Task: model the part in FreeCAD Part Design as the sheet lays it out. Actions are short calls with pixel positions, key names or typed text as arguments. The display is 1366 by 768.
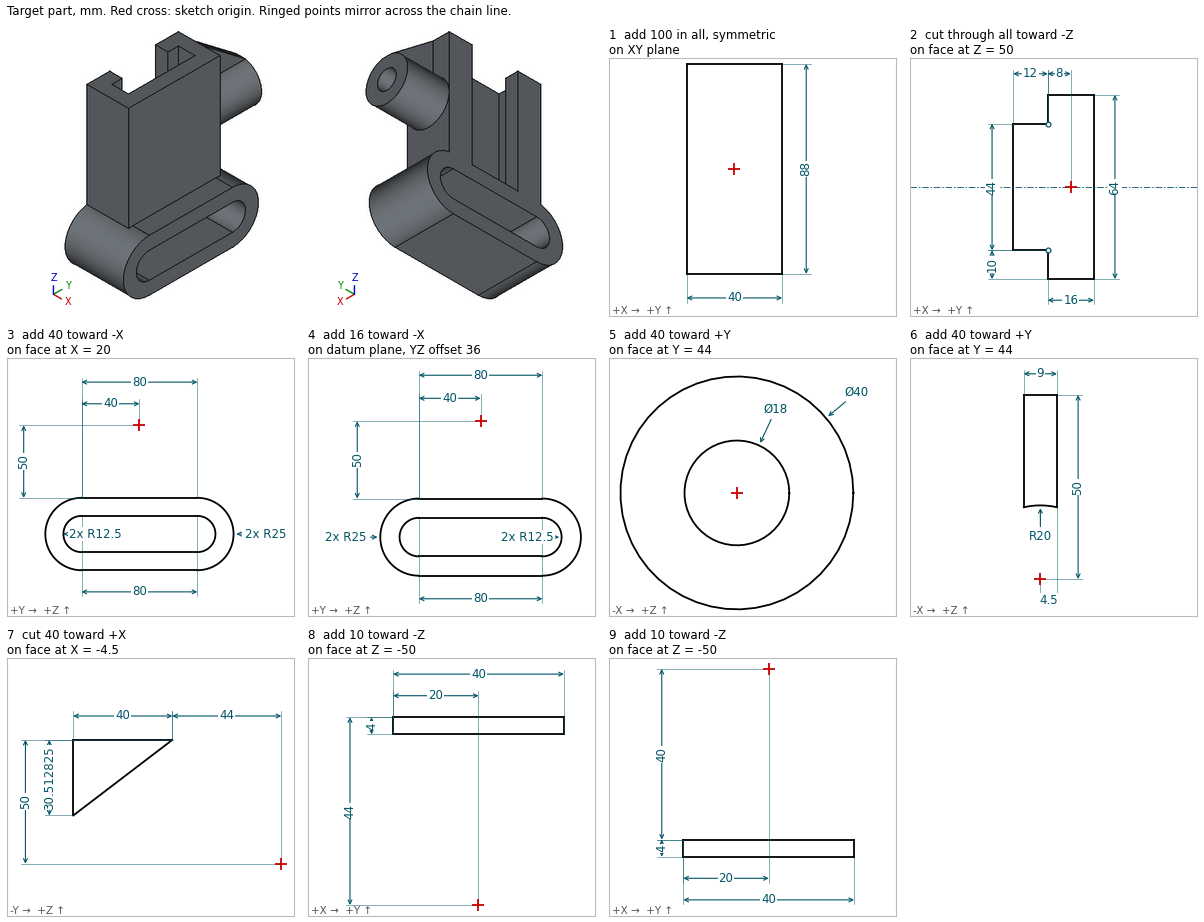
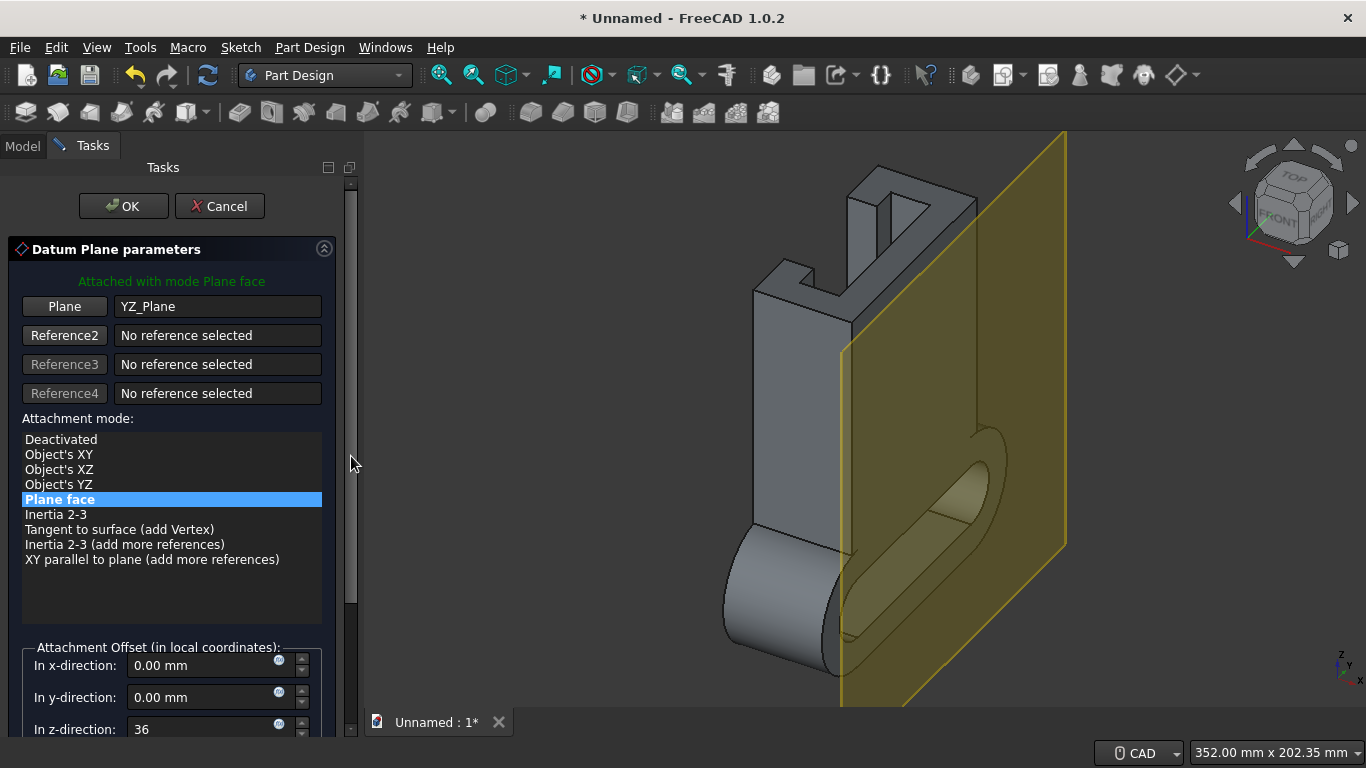
click(124, 206)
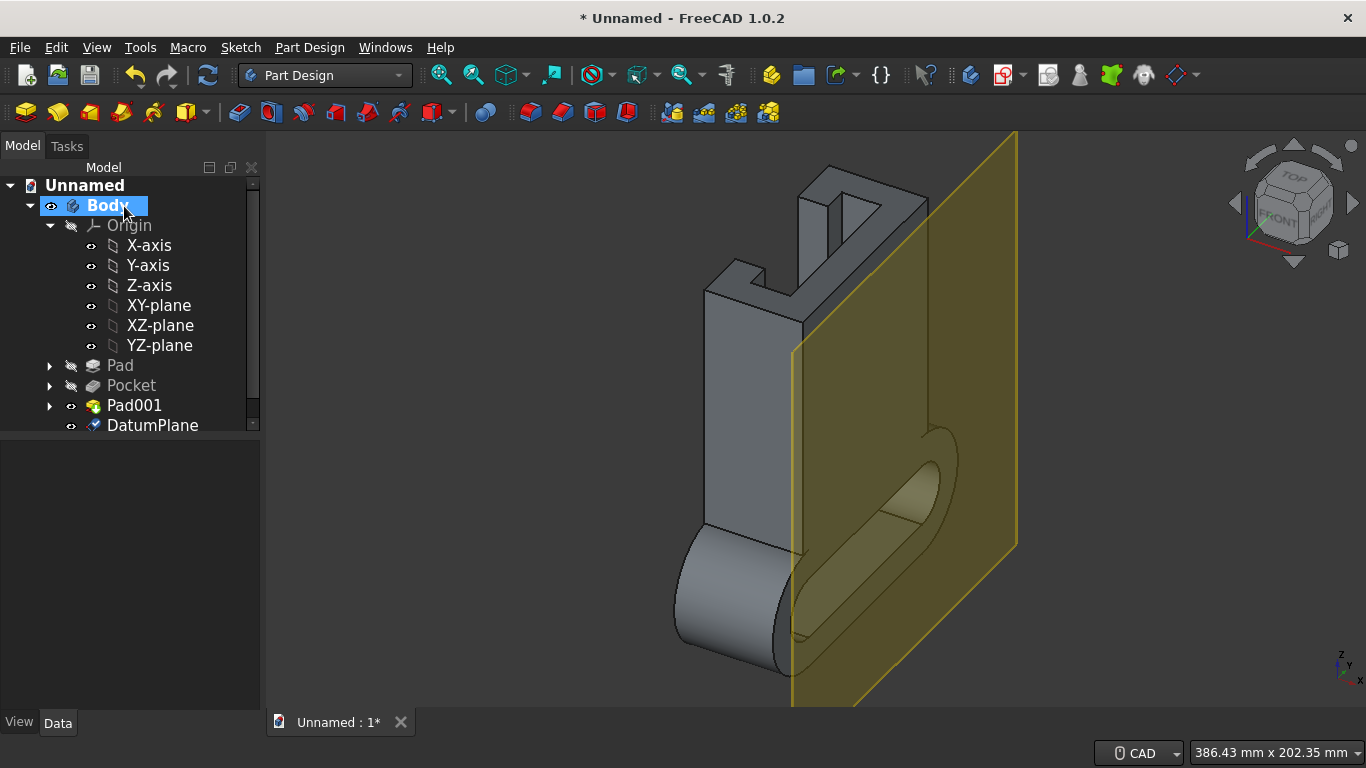
click(116, 426)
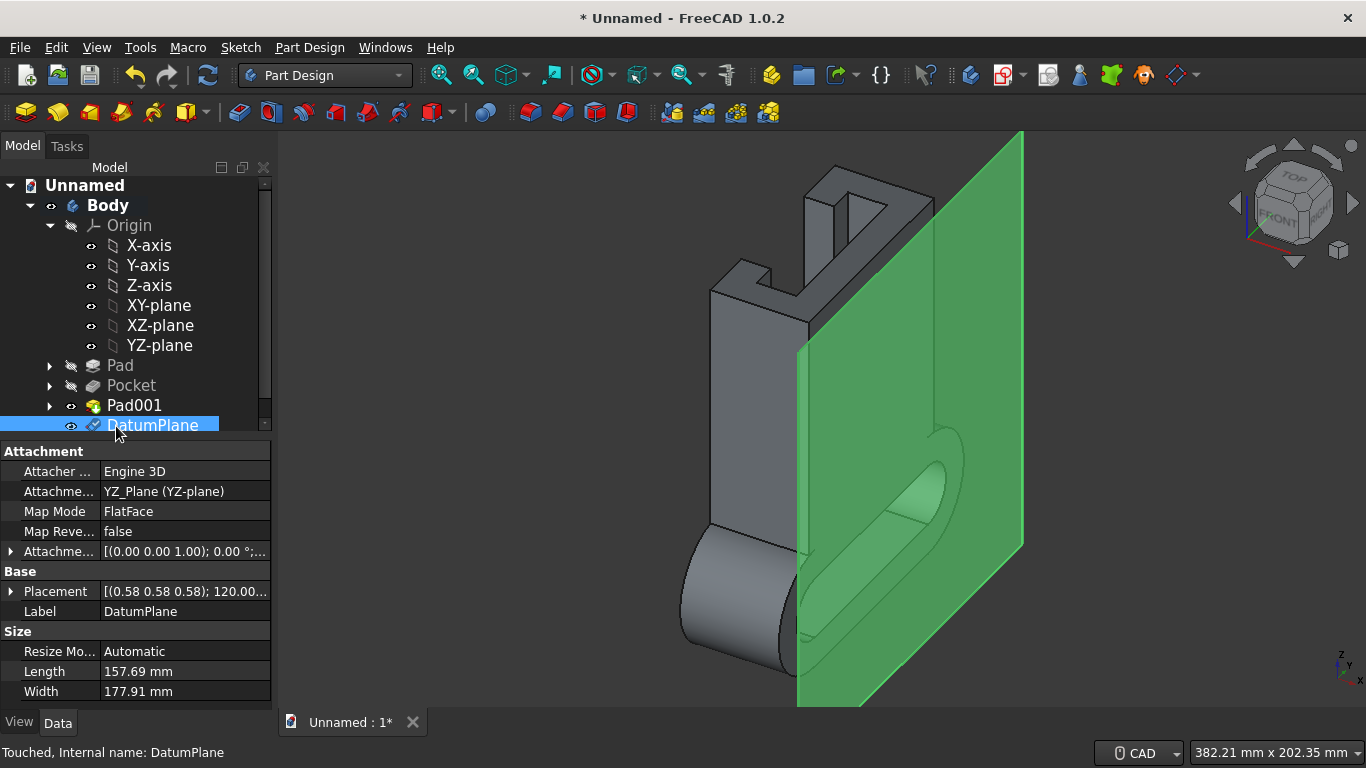
click(1004, 76)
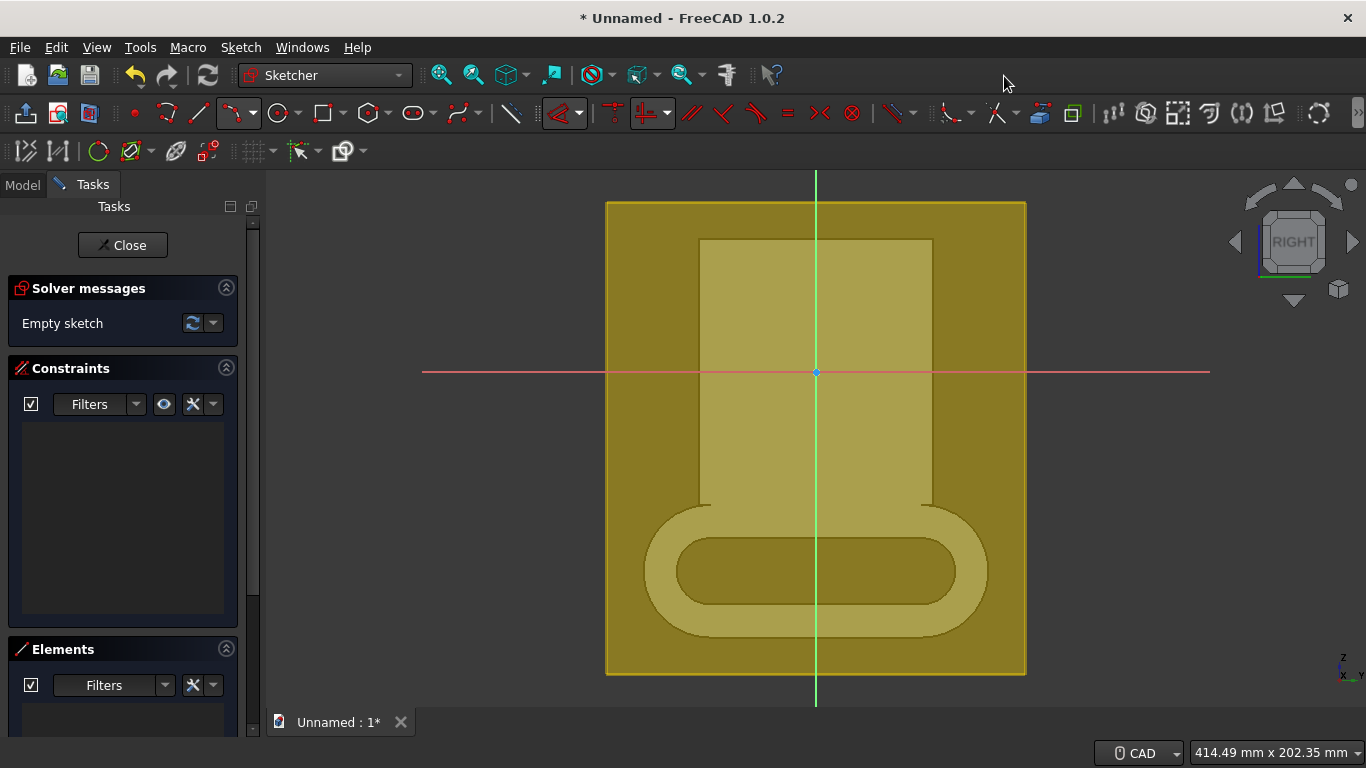
key(g)
key(s)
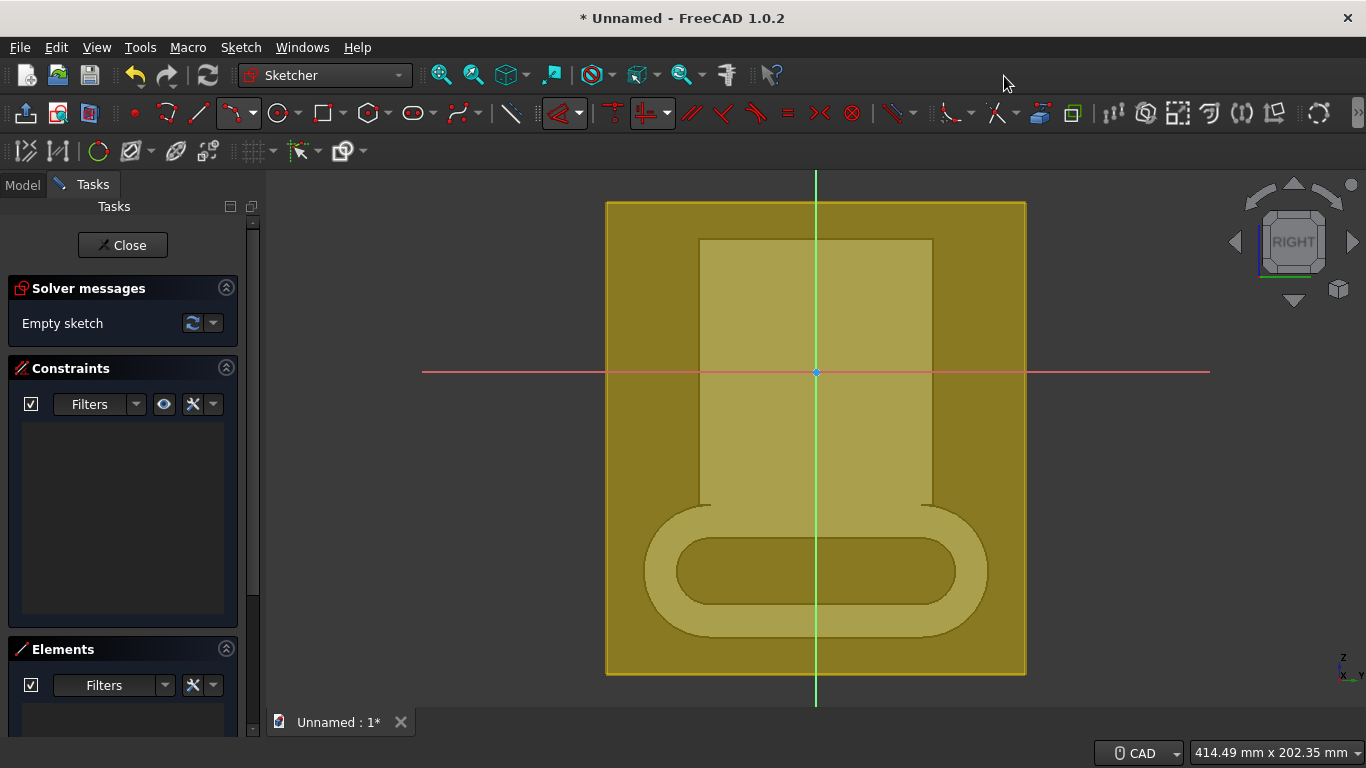
click(710, 571)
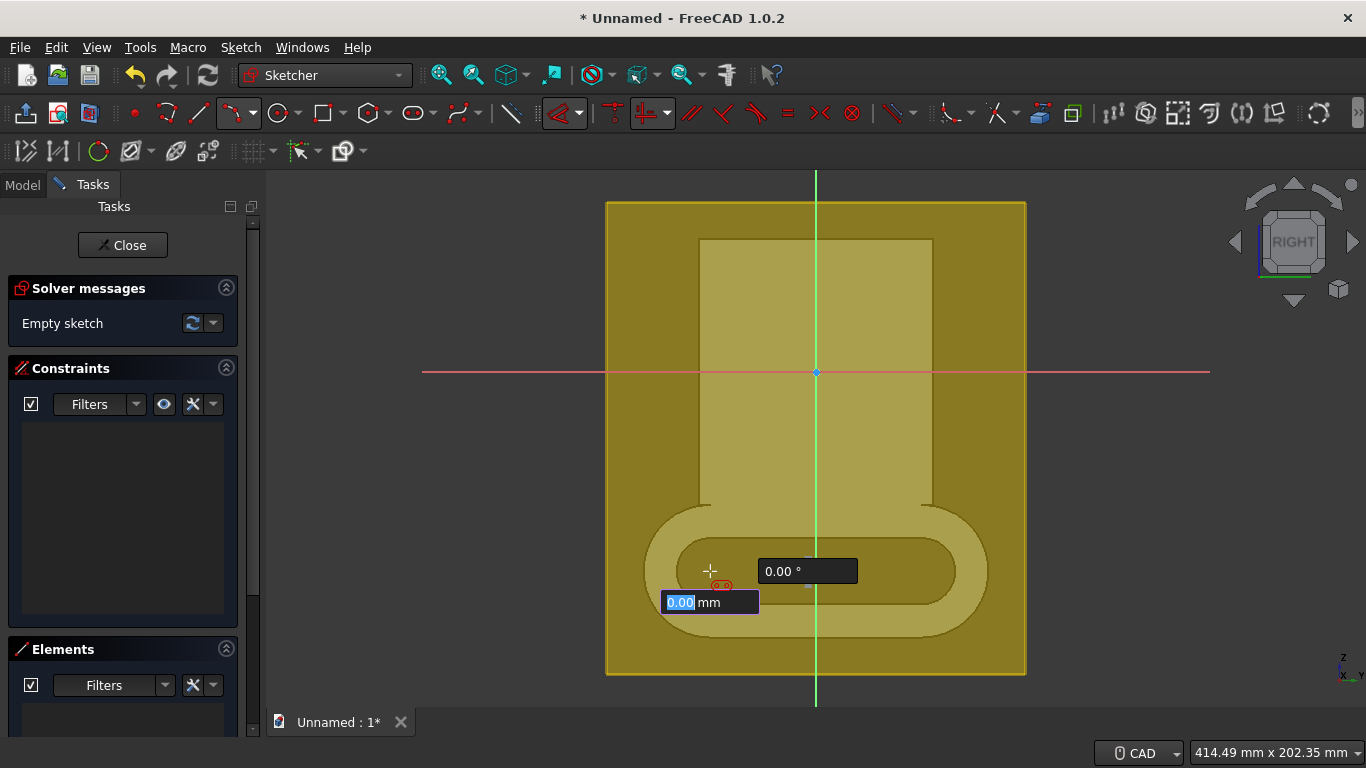
click(922, 571)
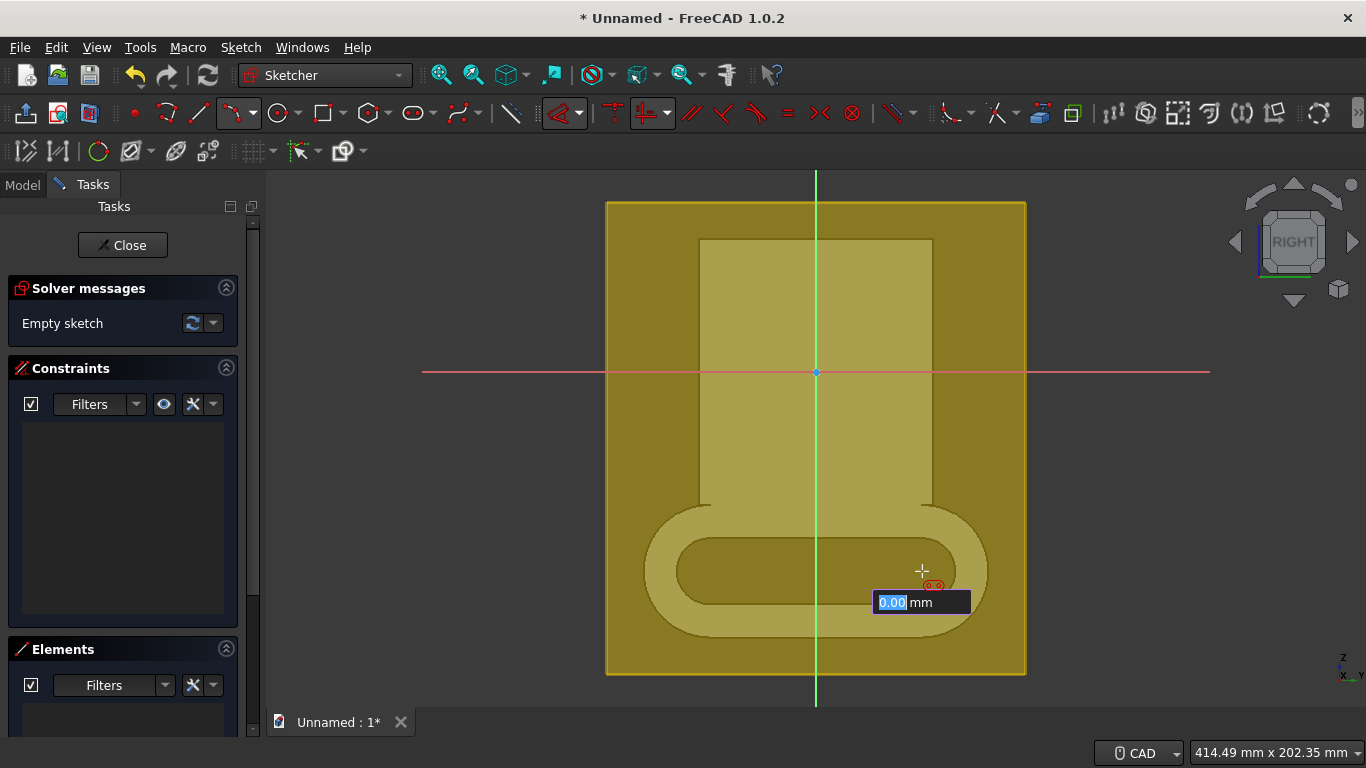
click(848, 505)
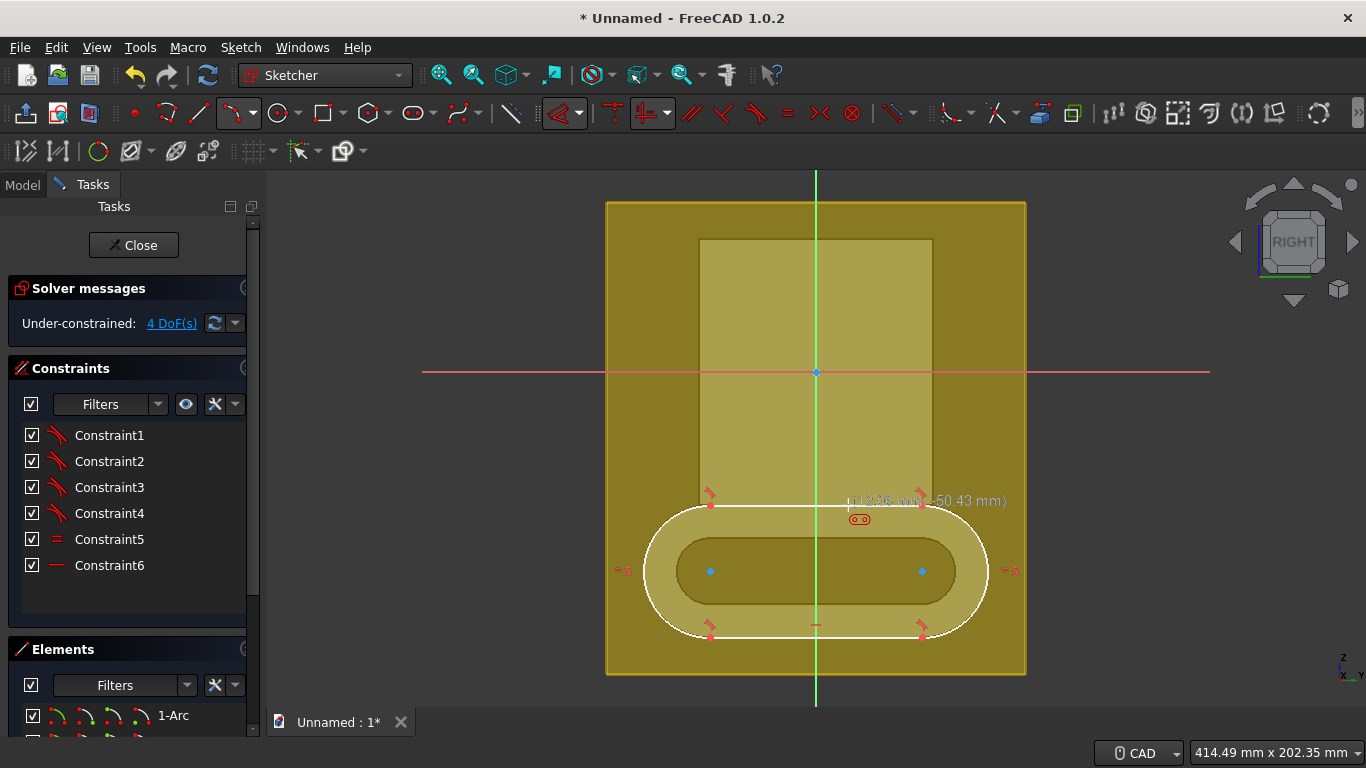
click(710, 572)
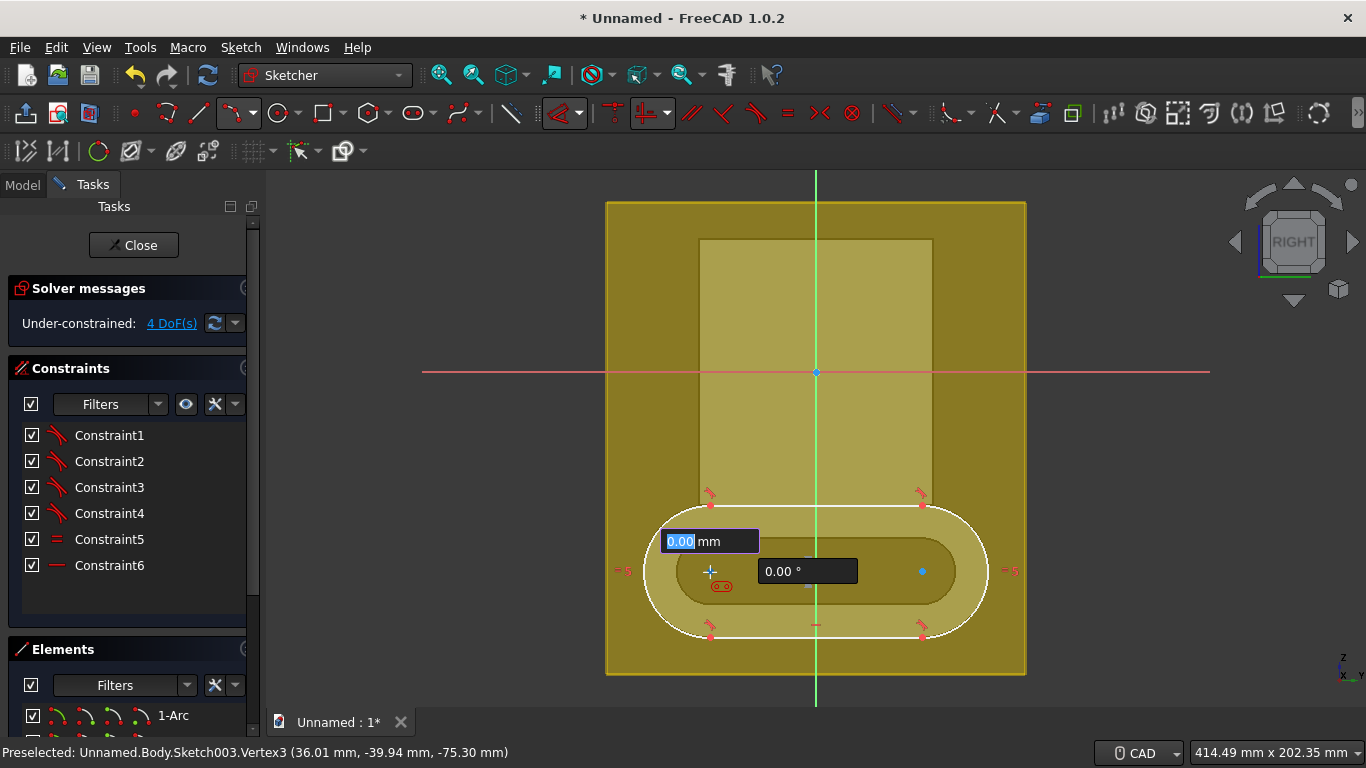
click(922, 572)